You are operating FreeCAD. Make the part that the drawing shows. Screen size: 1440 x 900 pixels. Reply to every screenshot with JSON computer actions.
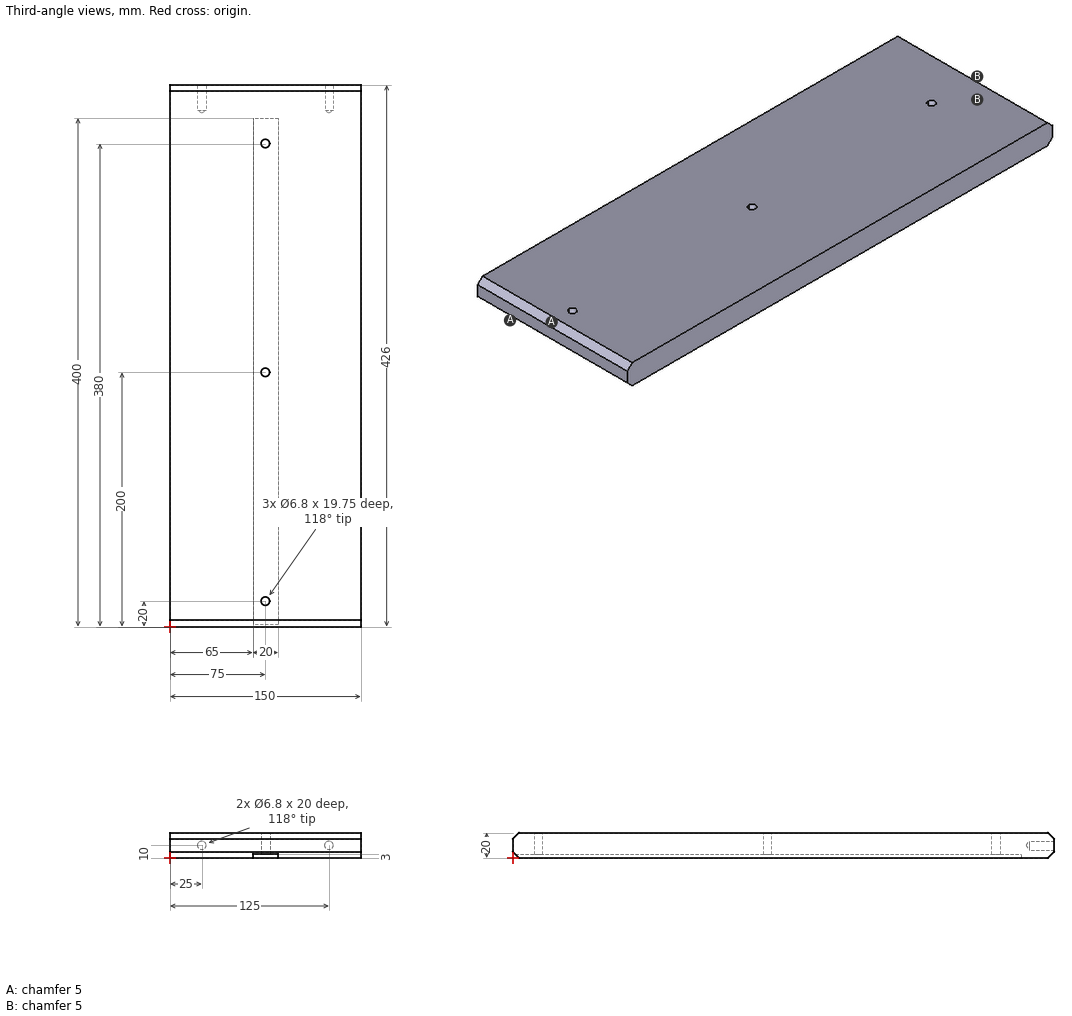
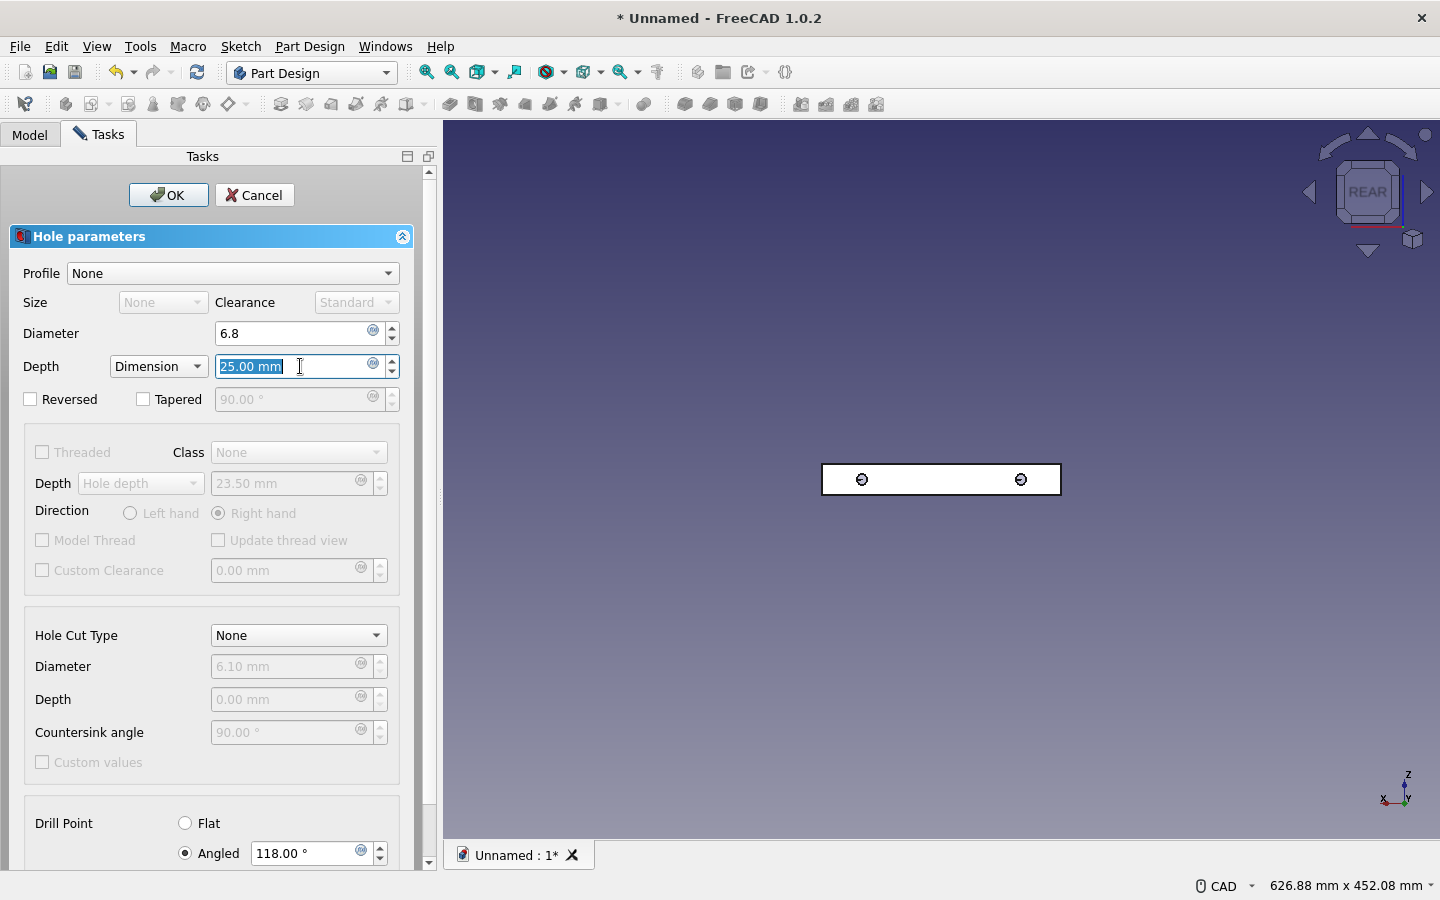
{"action": "type", "text": "20"}
{"action": "key", "text": "Tab"}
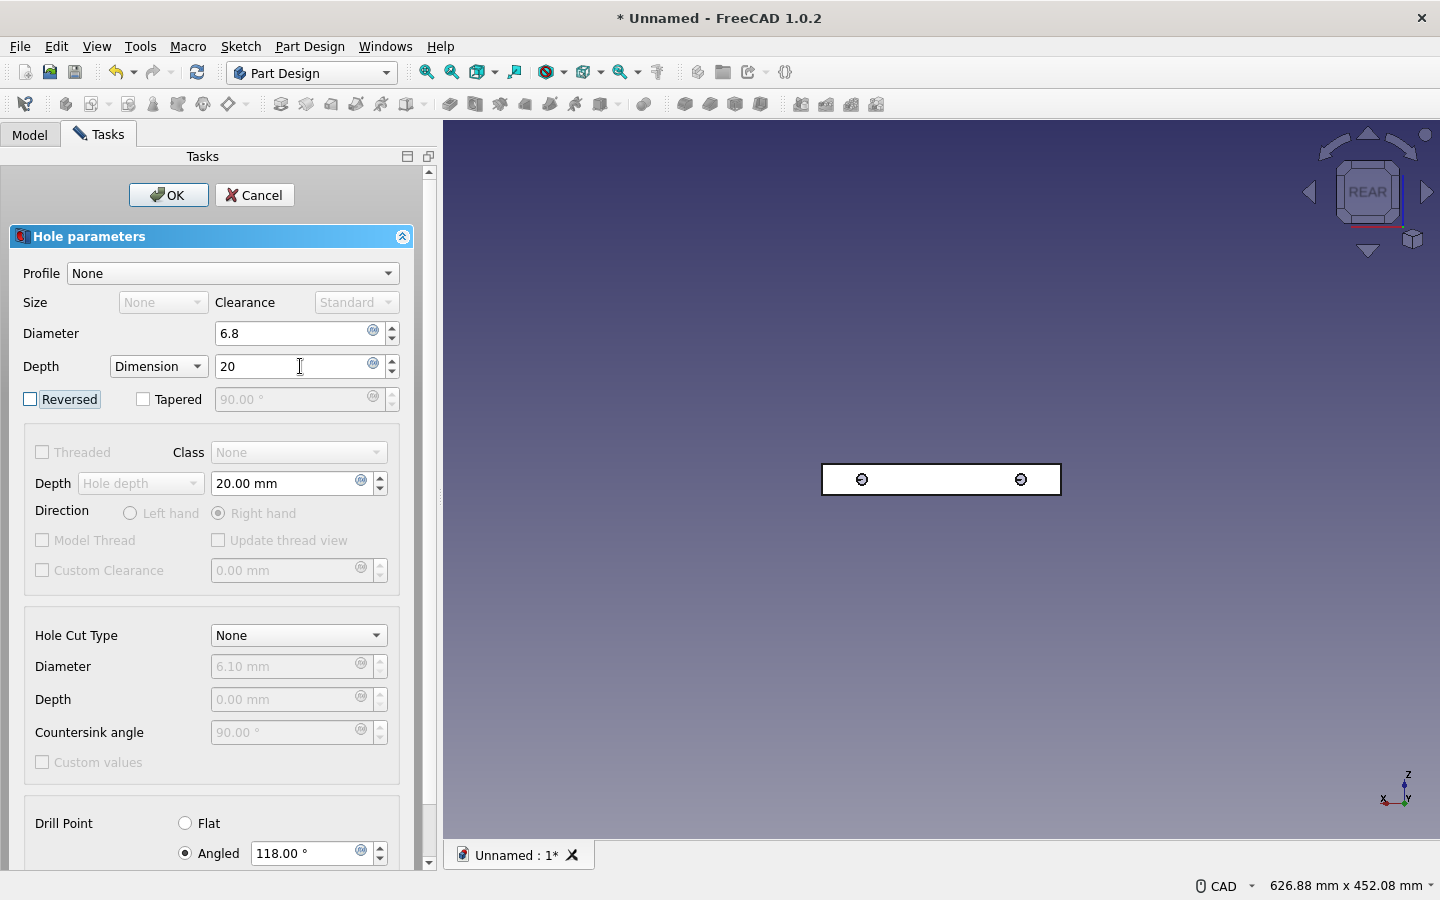
{"action": "left_click", "coordinate": [169, 195]}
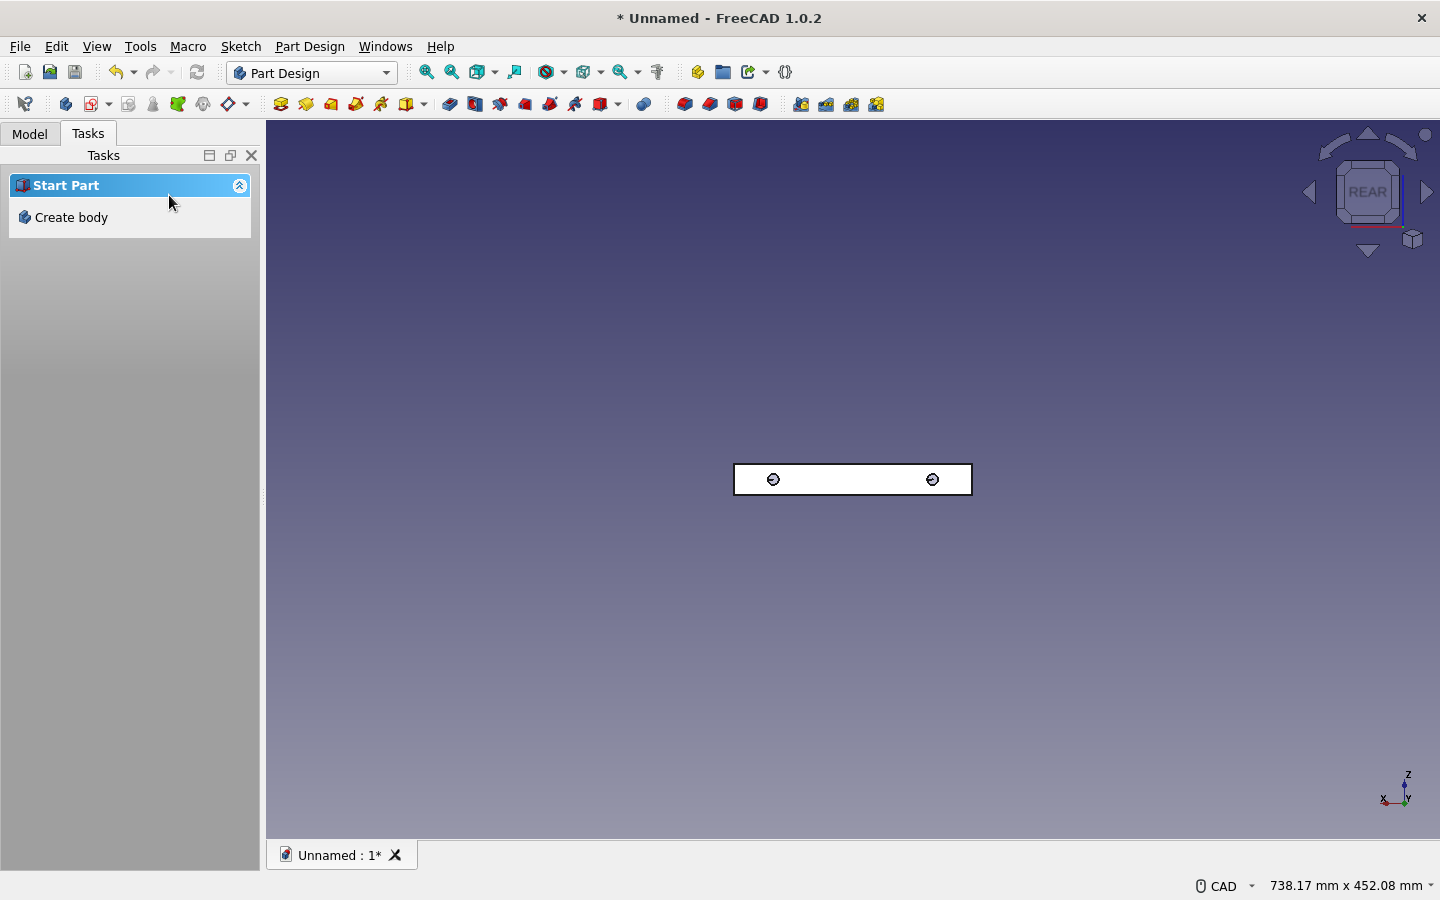
{"action": "left_click", "coordinate": [427, 72]}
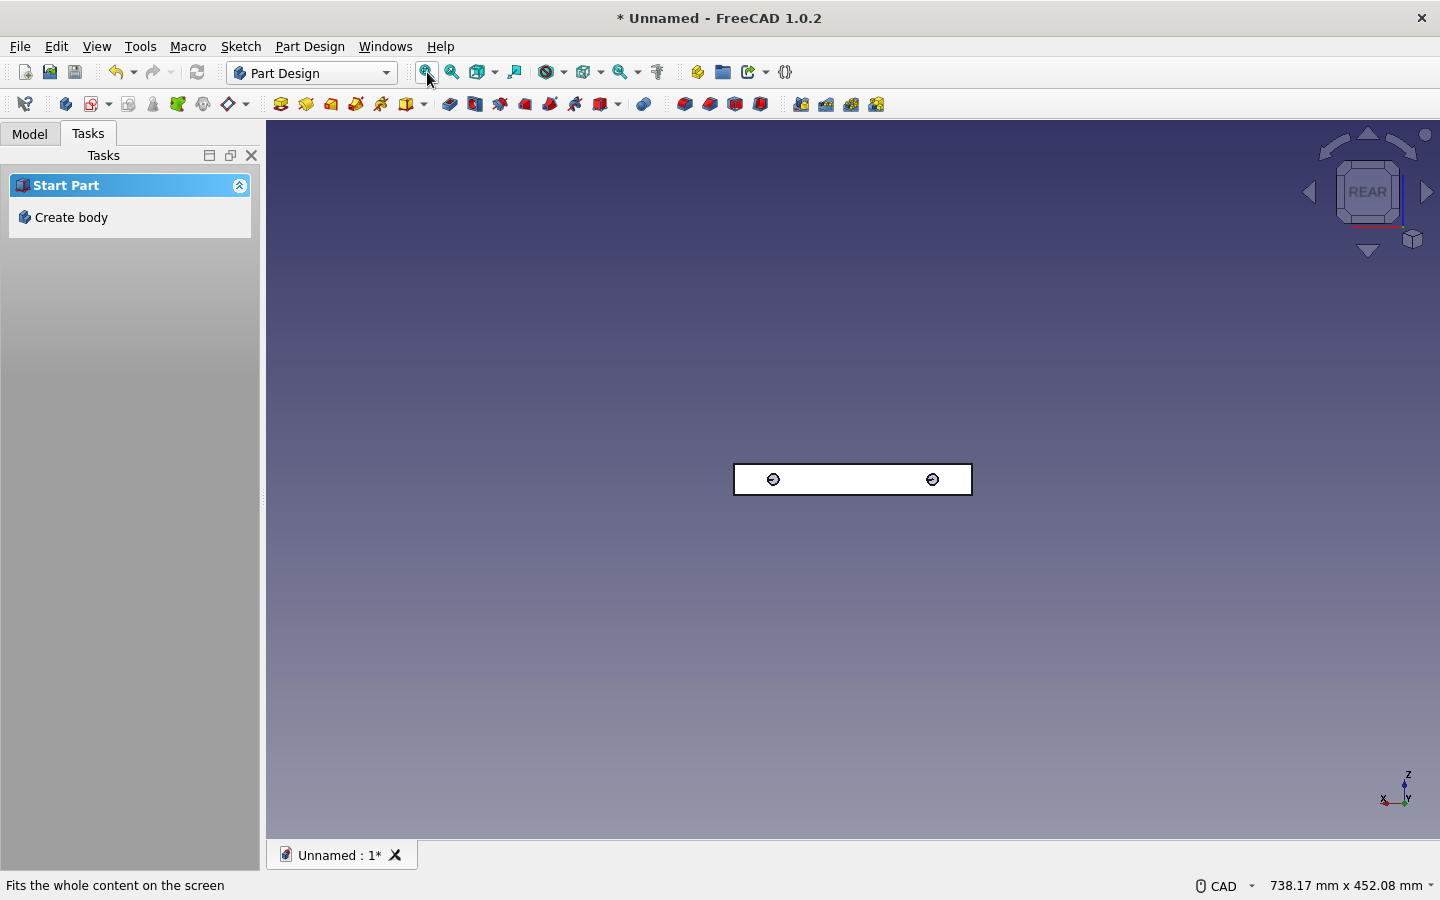
{"action": "key", "text": "0"}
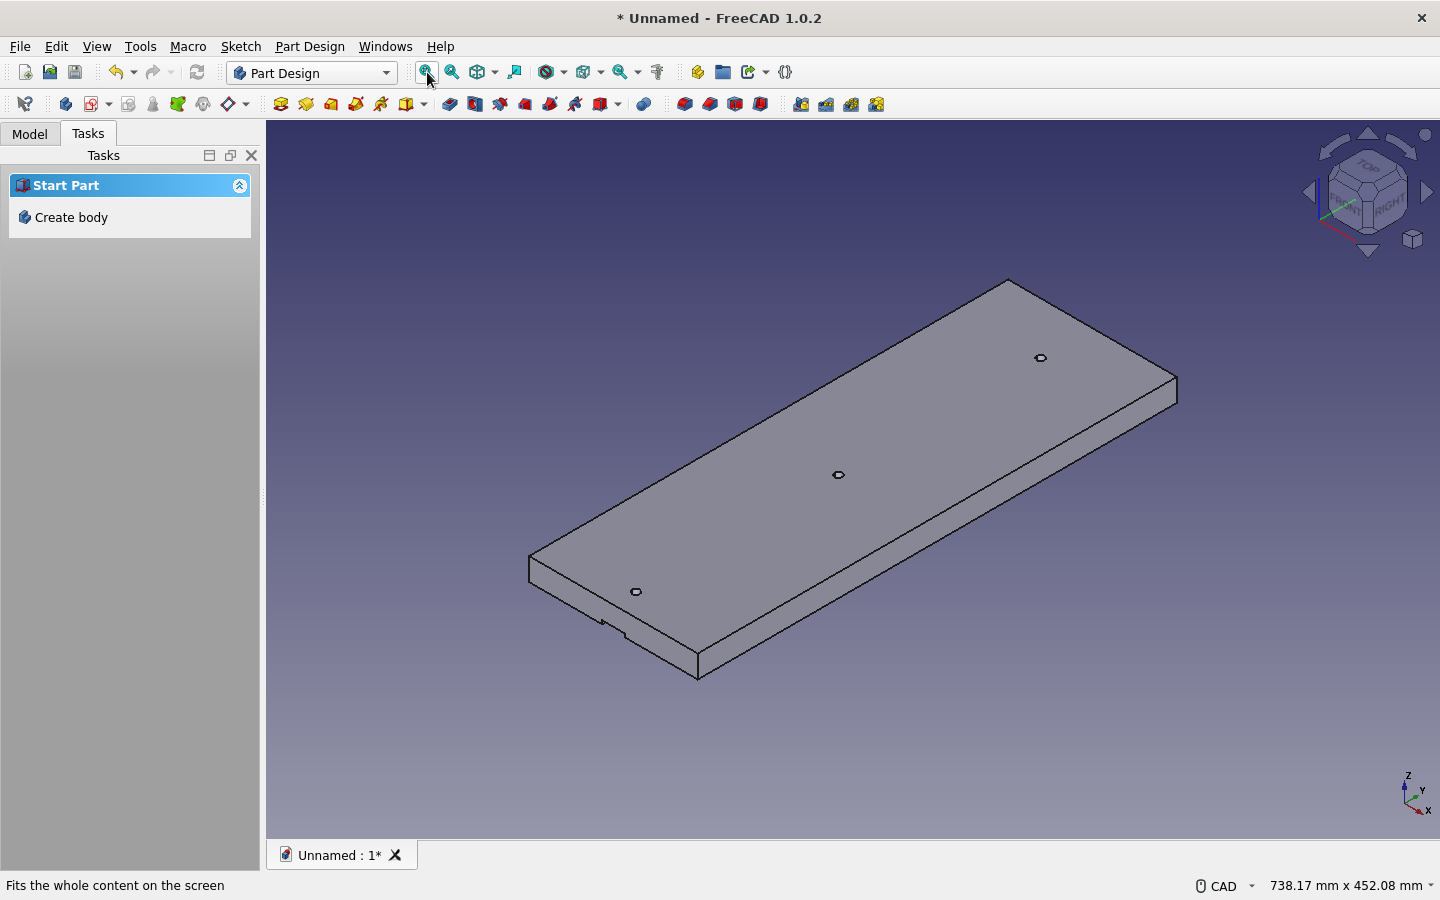
{"action": "left_click", "coordinate": [613, 604]}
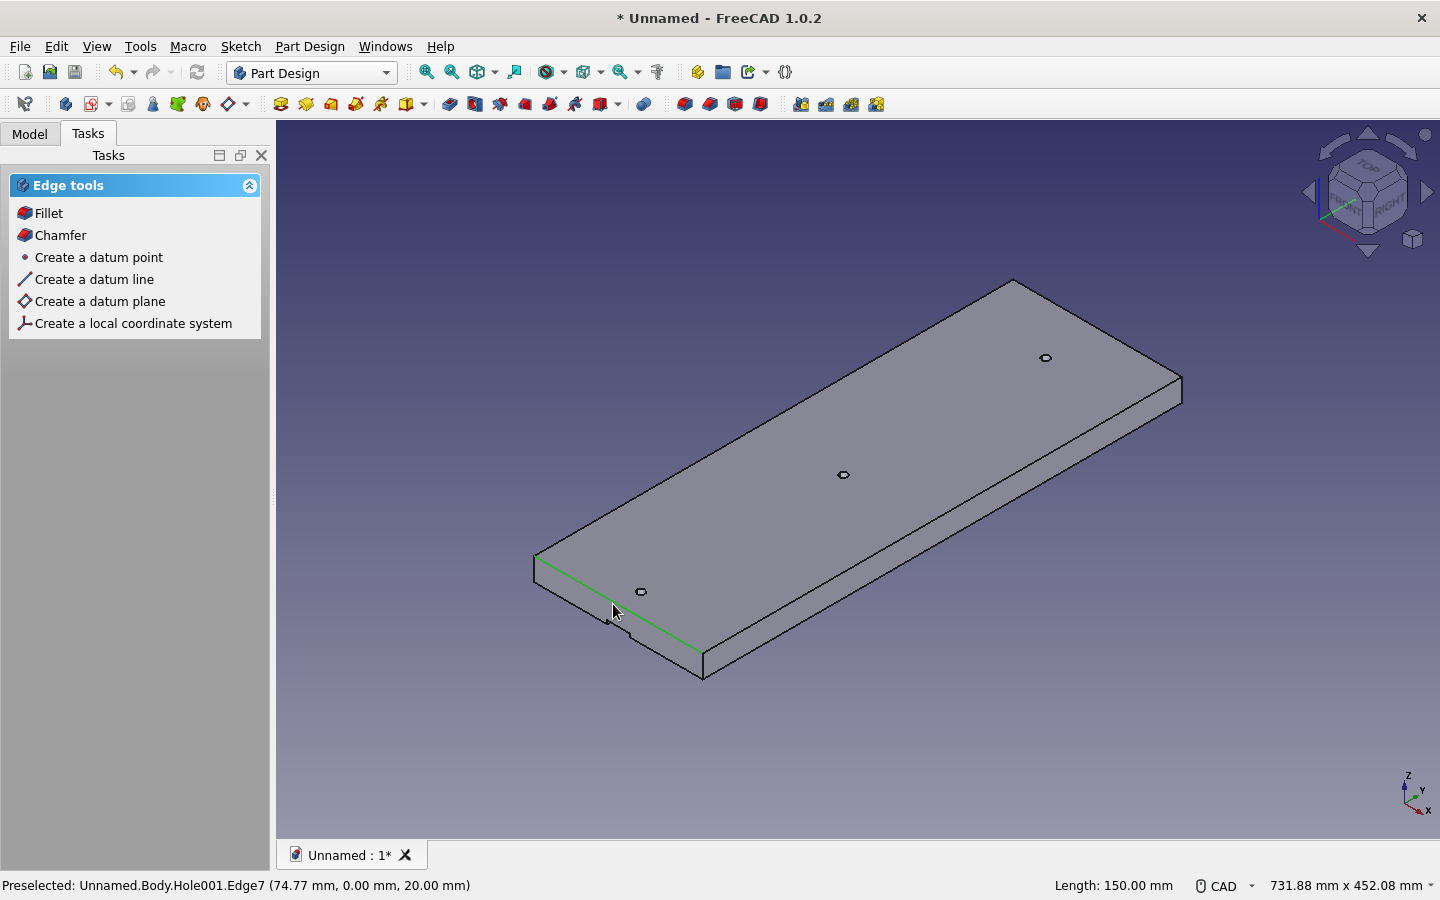
{"action": "key", "text": "2"}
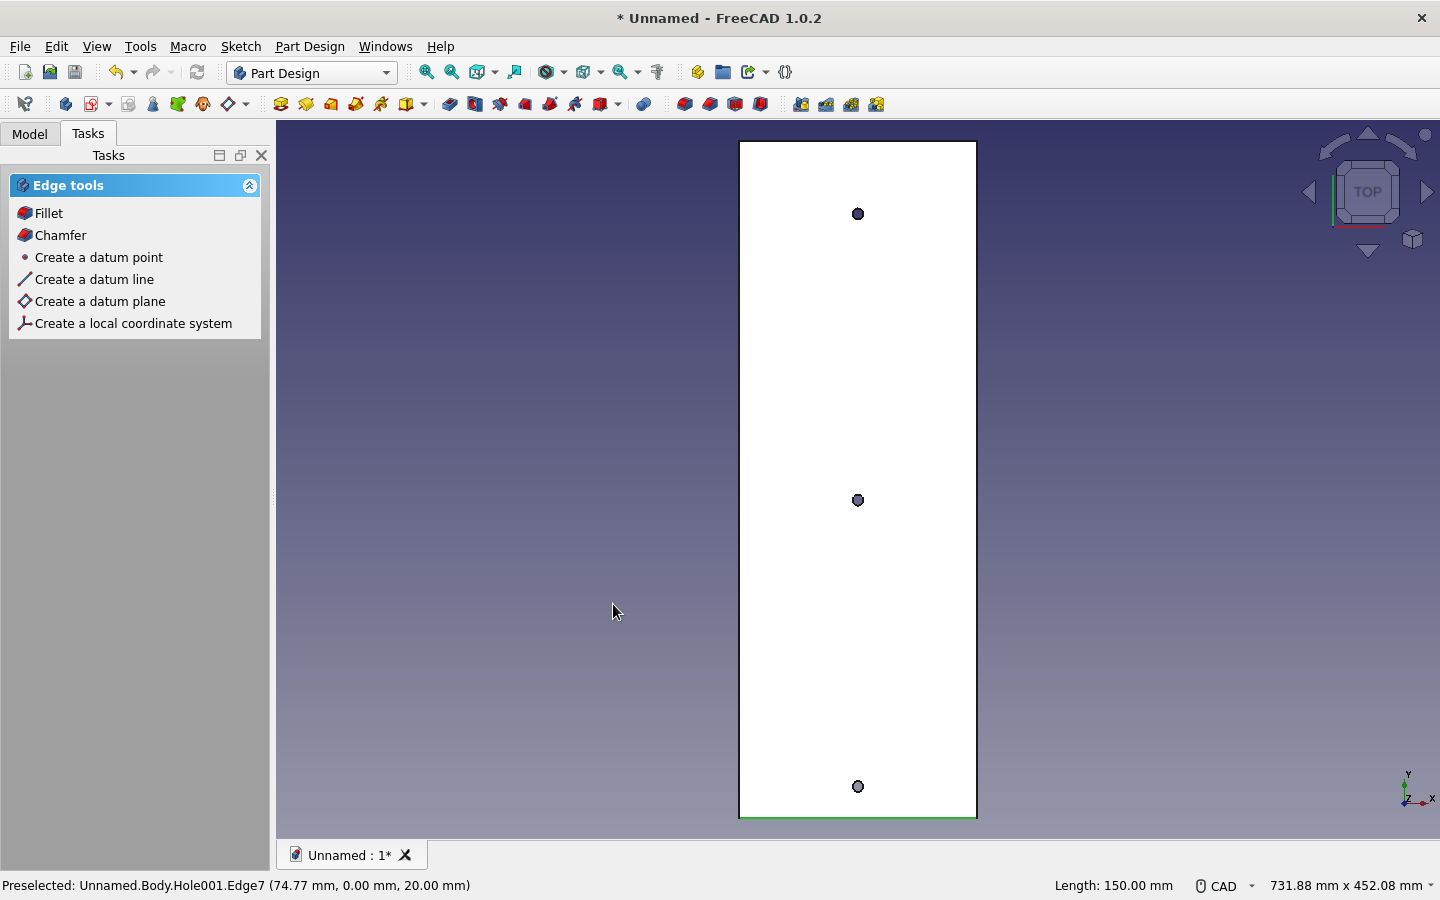
{"action": "key", "text": "1"}